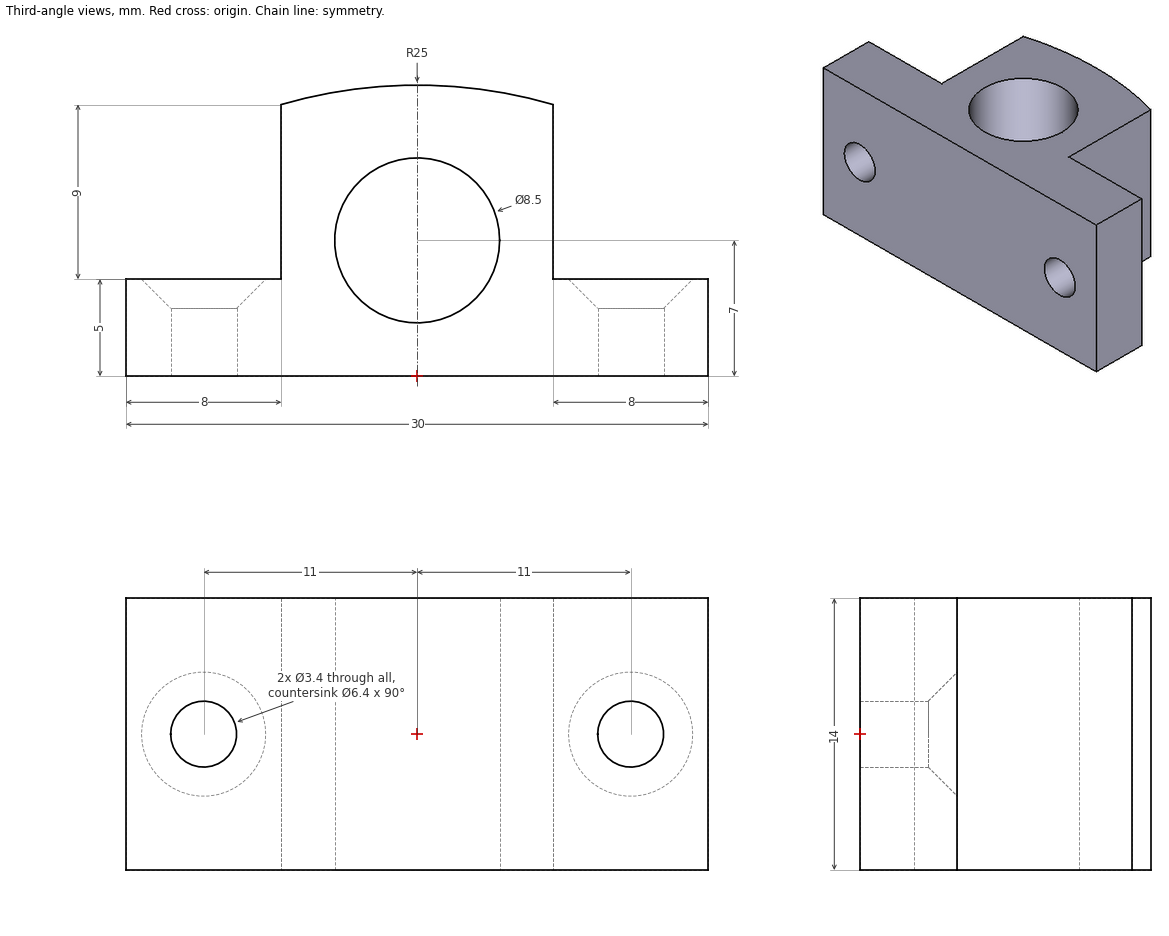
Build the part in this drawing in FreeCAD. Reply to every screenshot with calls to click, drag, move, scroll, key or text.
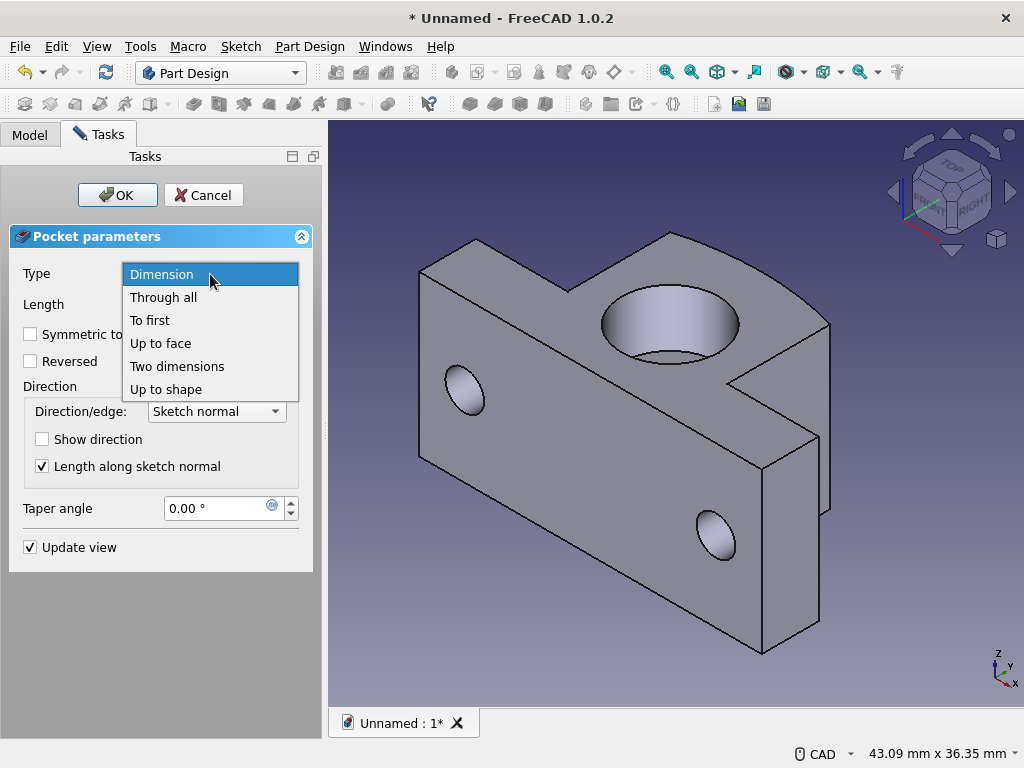
click(208, 298)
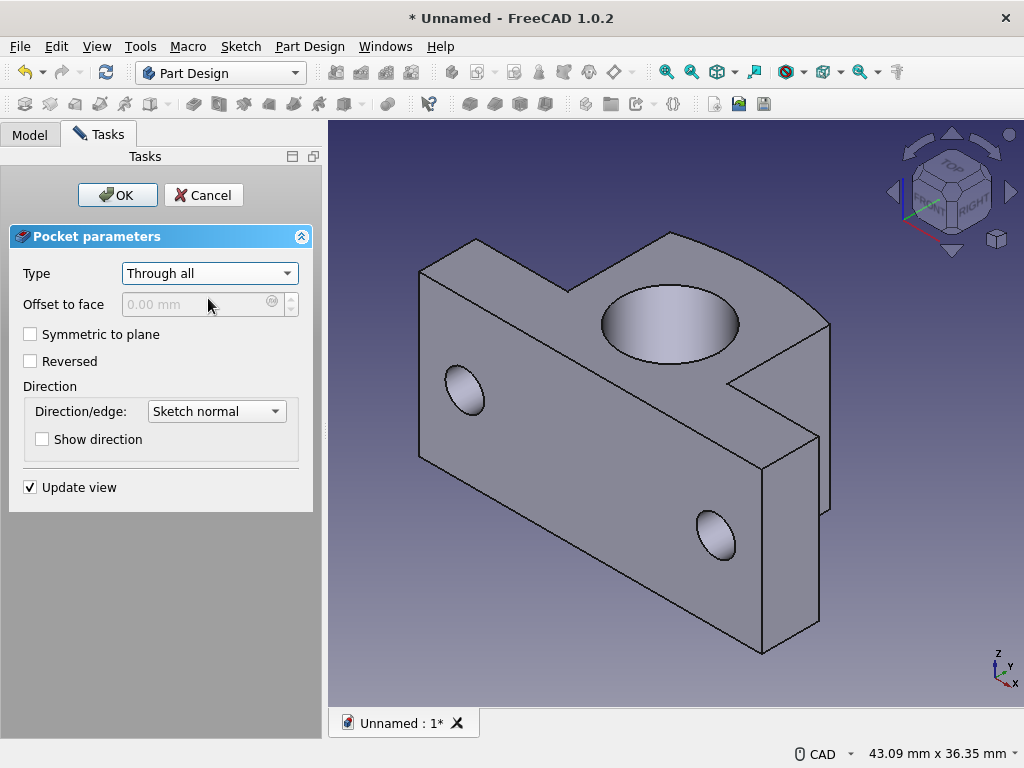
click(118, 195)